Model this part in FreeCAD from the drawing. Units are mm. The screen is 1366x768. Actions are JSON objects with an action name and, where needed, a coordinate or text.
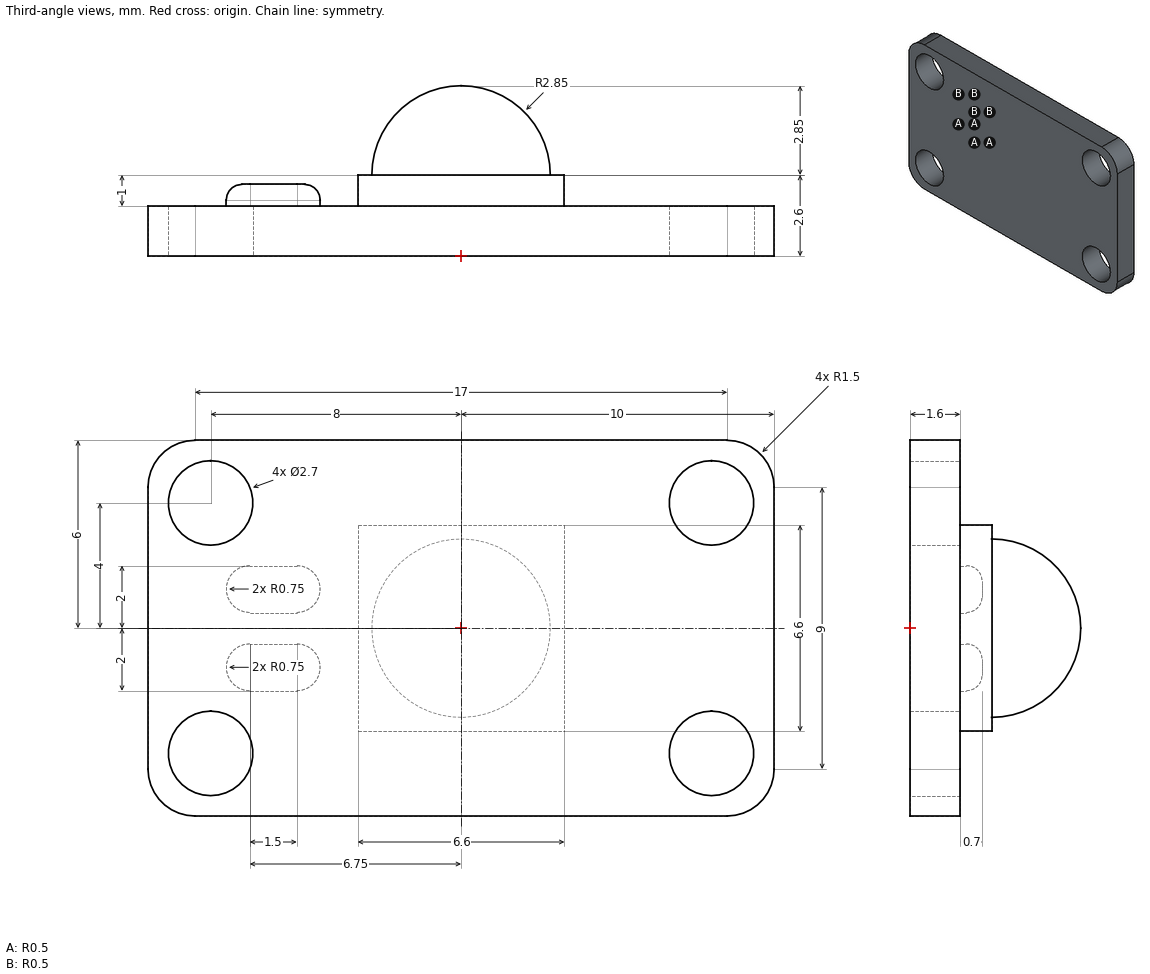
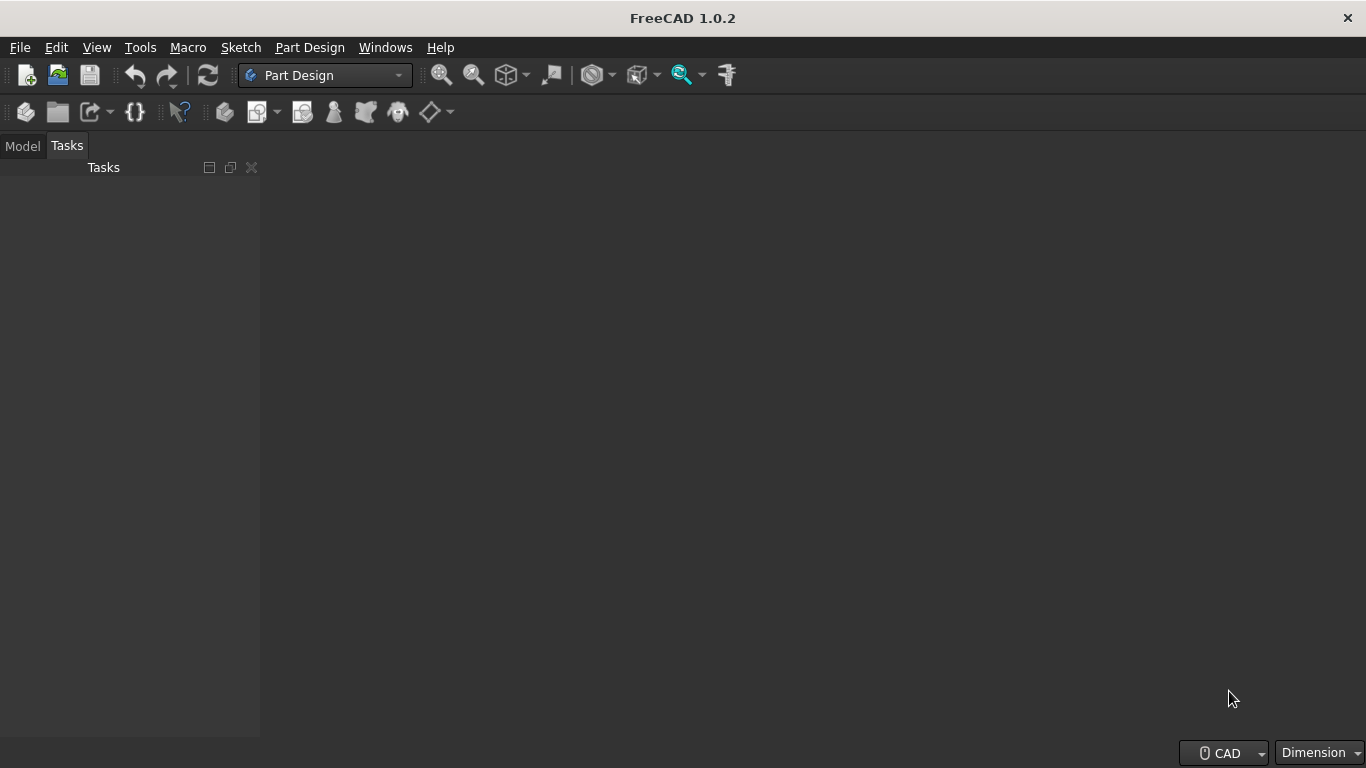
{"action": "left_click", "coordinate": [532, 112]}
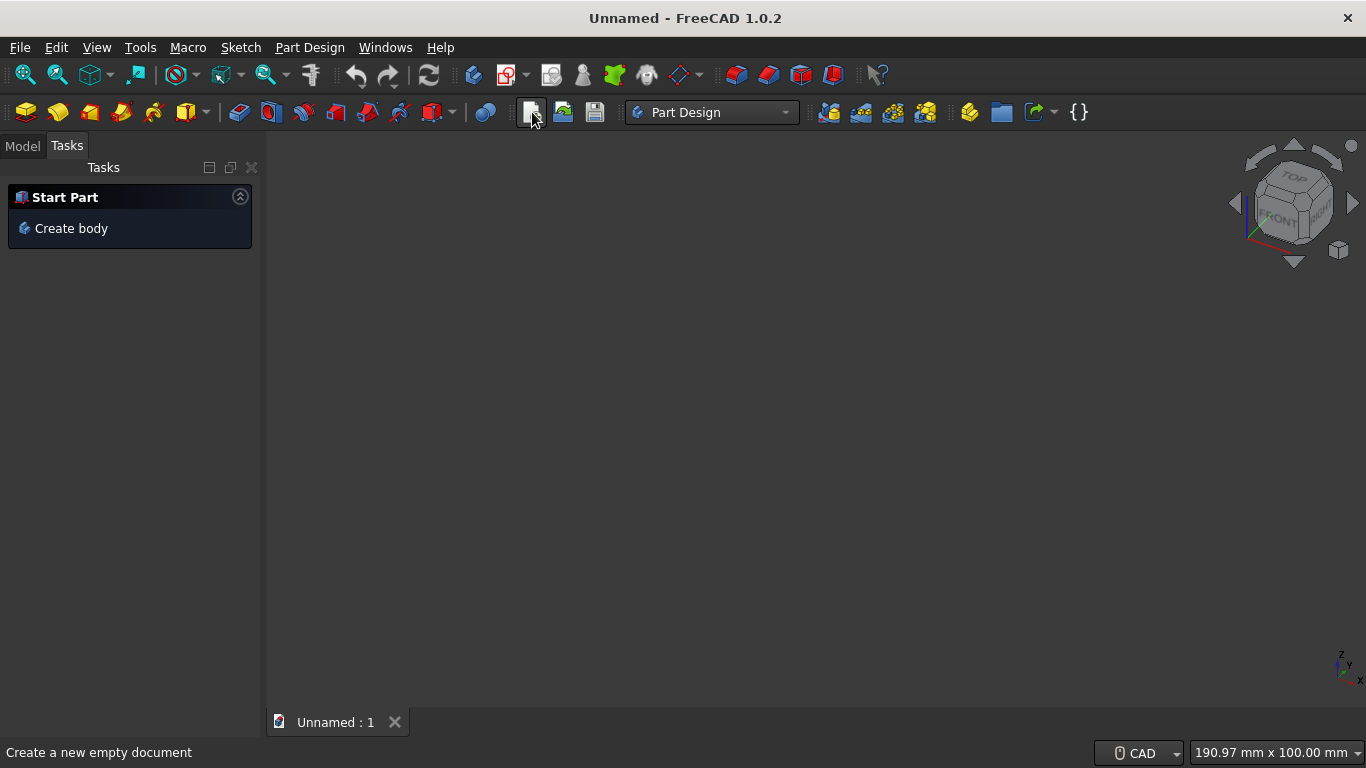
{"action": "left_click", "coordinate": [506, 76]}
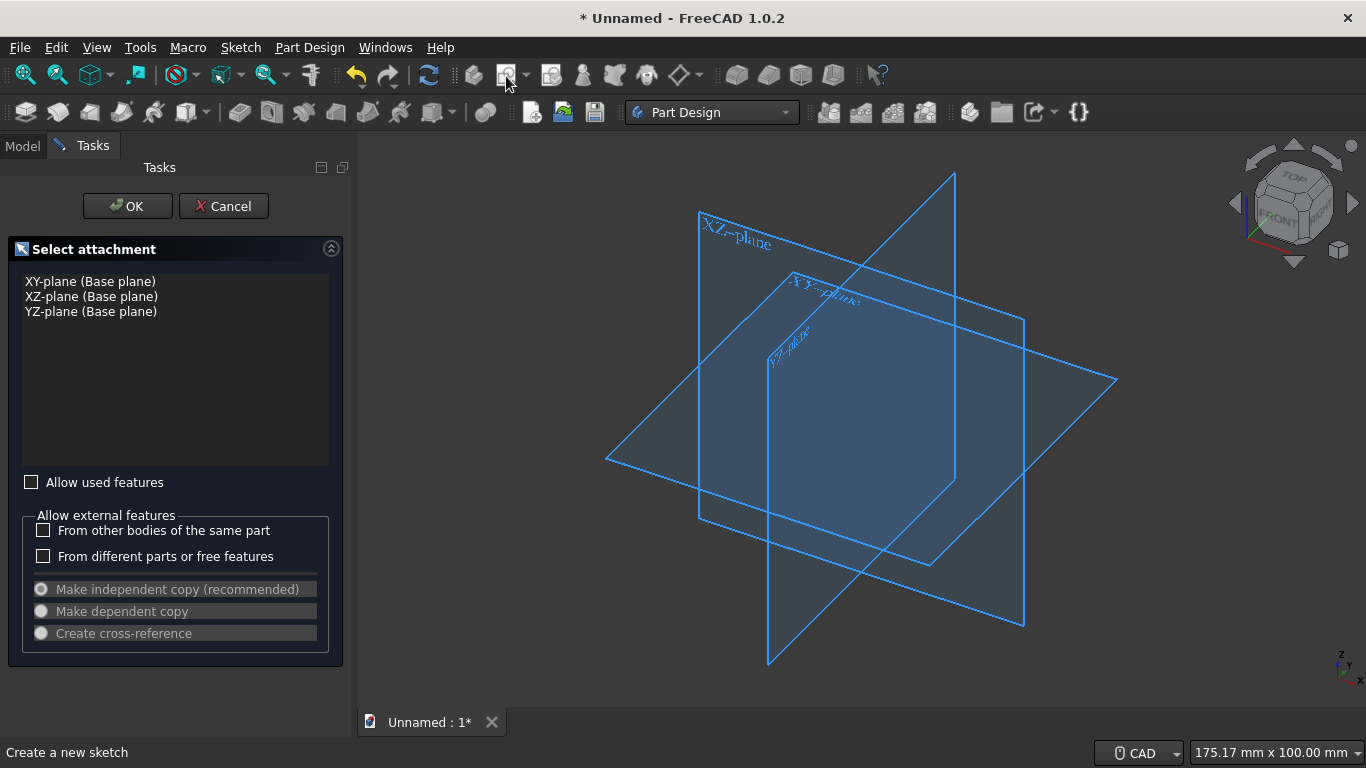
{"action": "left_click", "coordinate": [82, 296]}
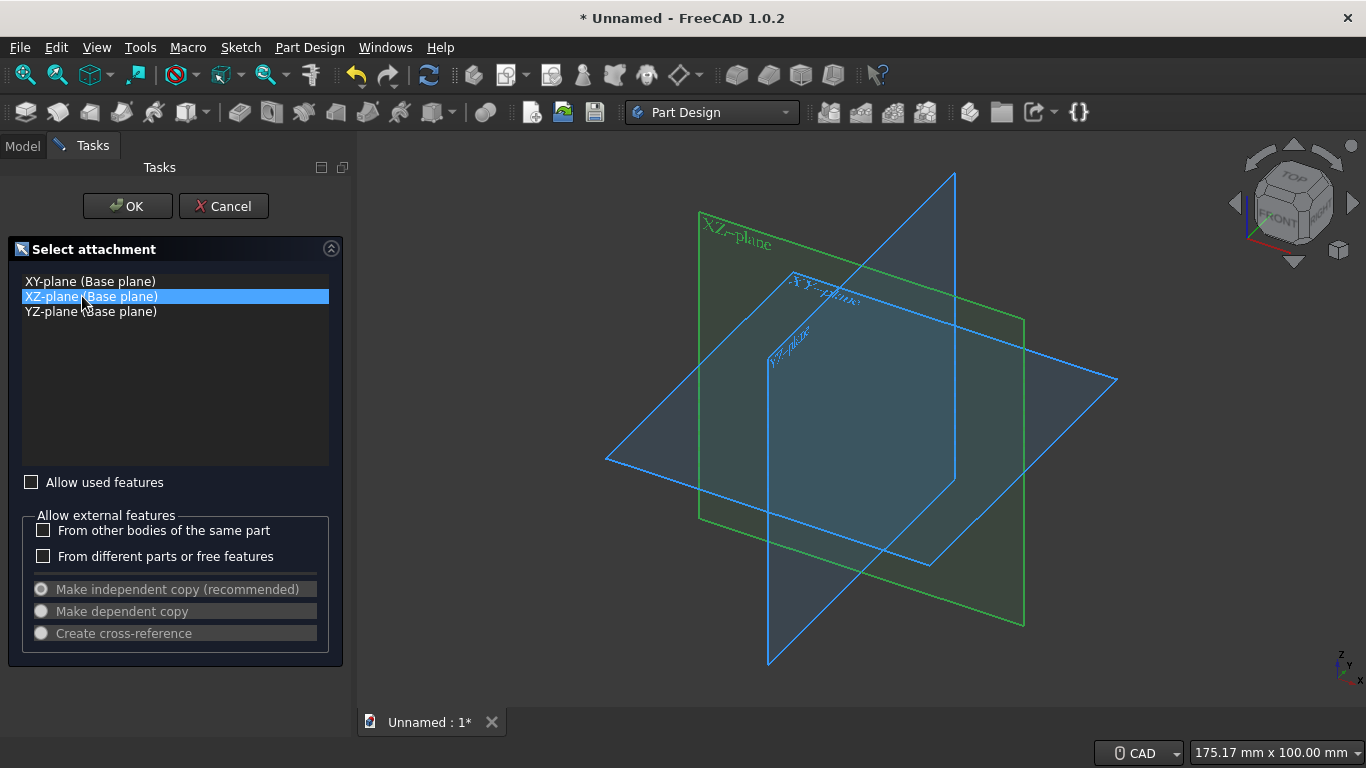
{"action": "left_click", "coordinate": [128, 206]}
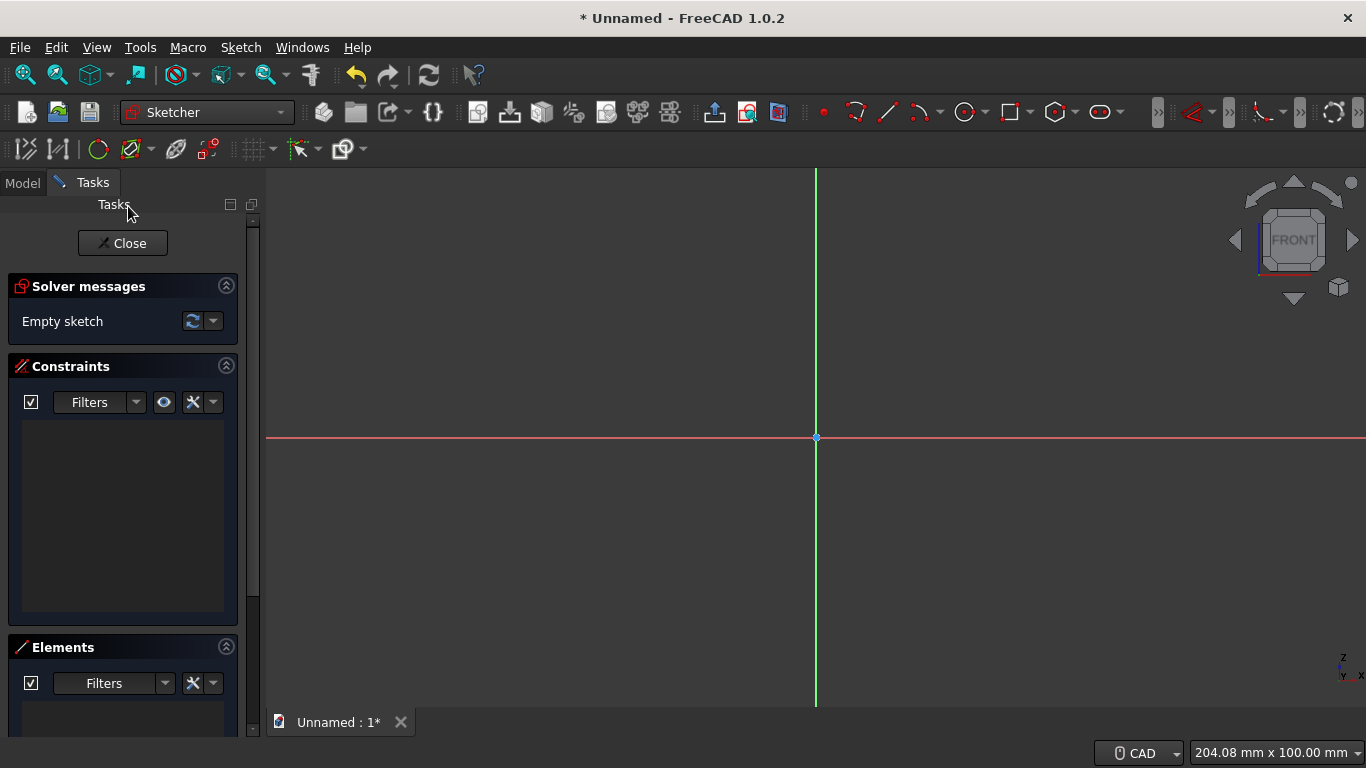
{"action": "scroll", "coordinate": [833, 438], "scroll_direction": "up", "scroll_amount": 8}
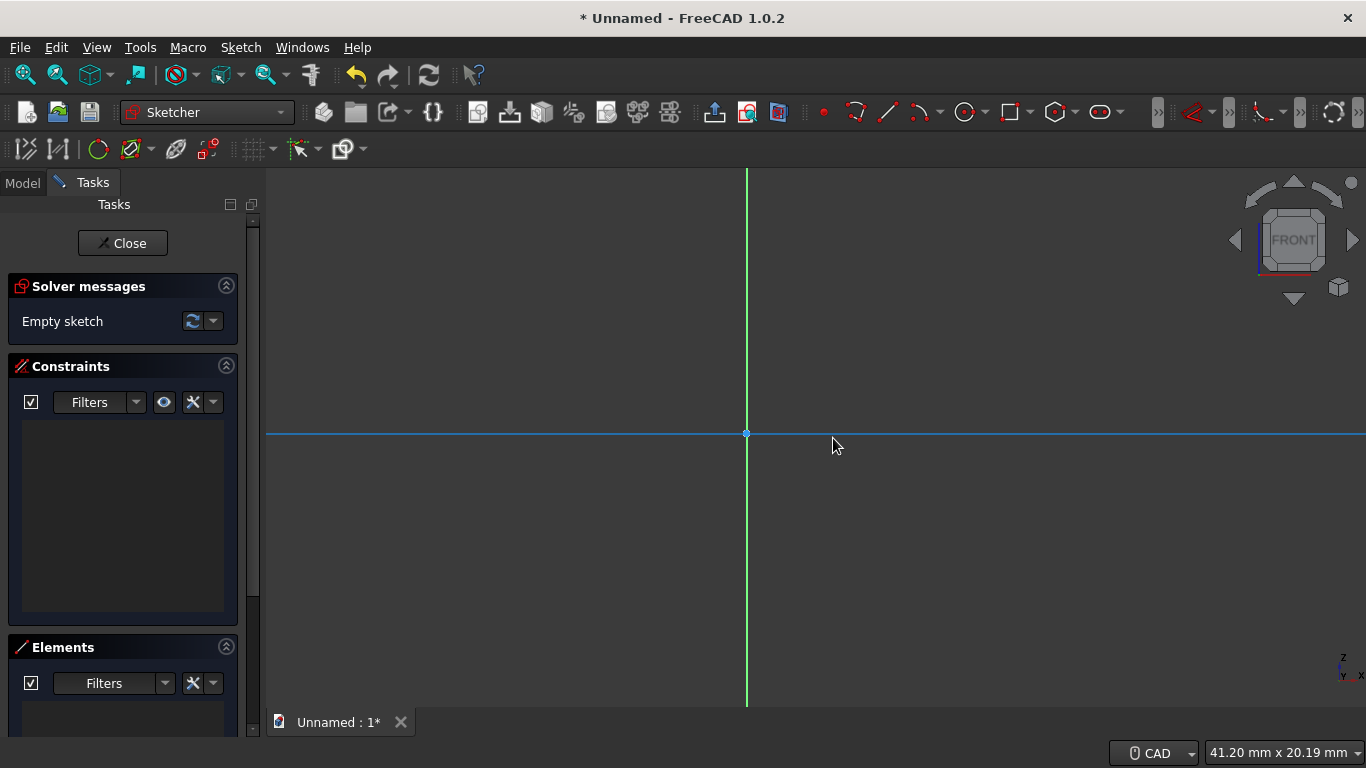
{"action": "left_click", "coordinate": [888, 112]}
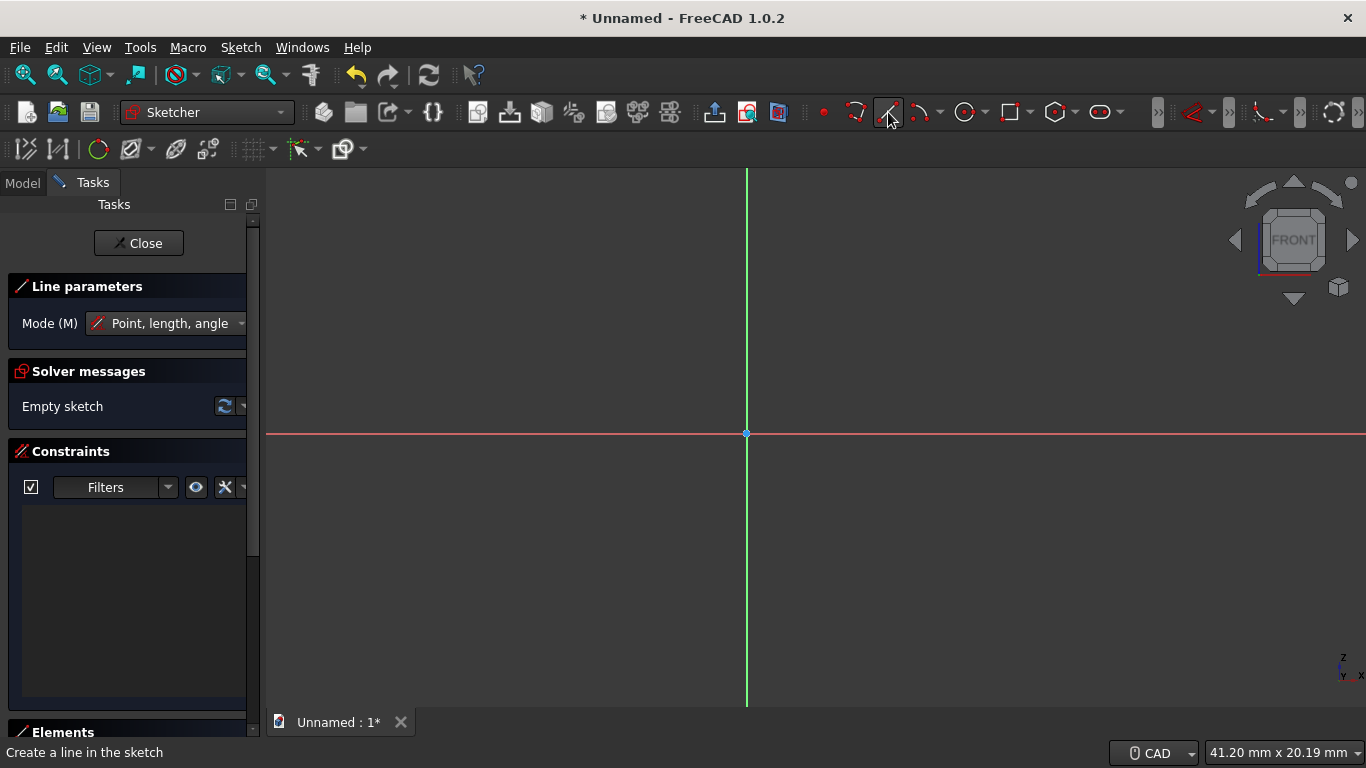
{"action": "left_click", "coordinate": [520, 273]}
{"action": "left_click", "coordinate": [974, 273]}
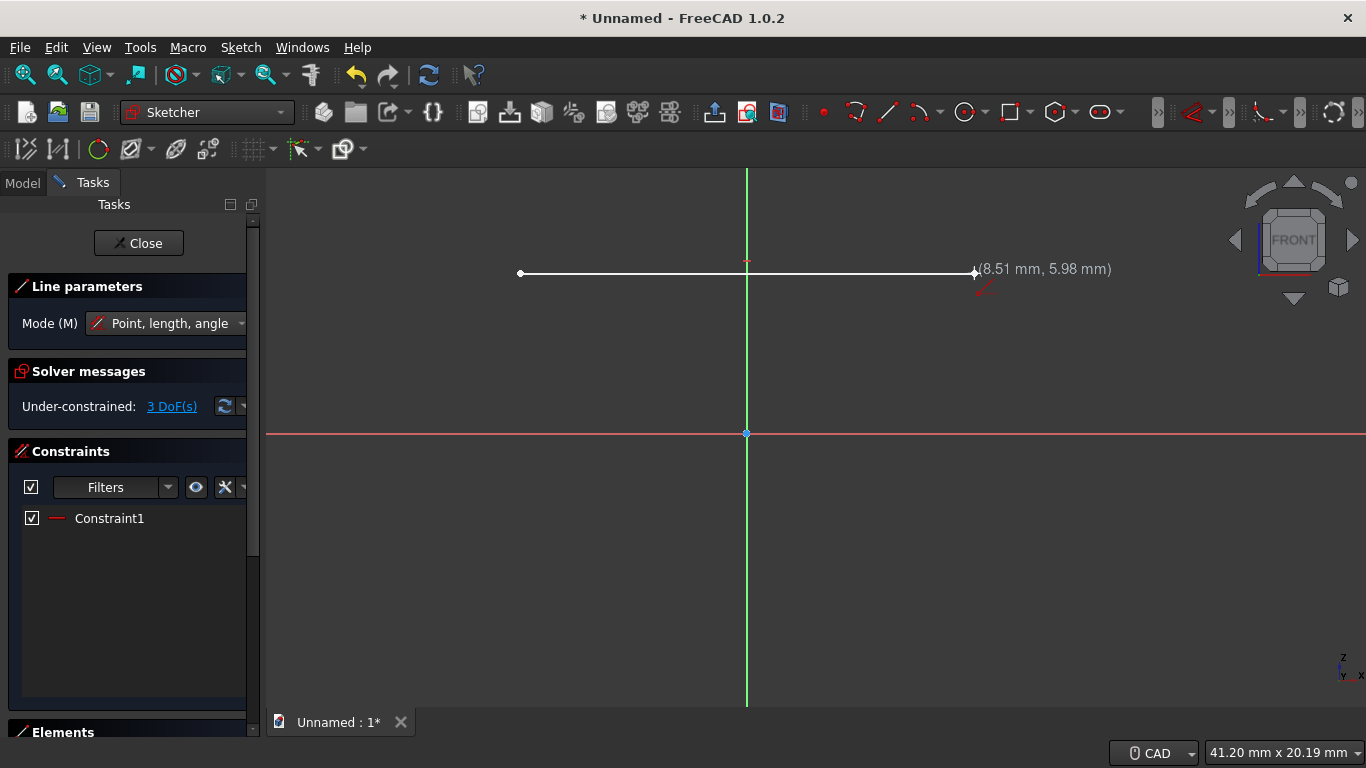
{"action": "left_click", "coordinate": [1014, 313]}
{"action": "left_click", "coordinate": [1014, 554]}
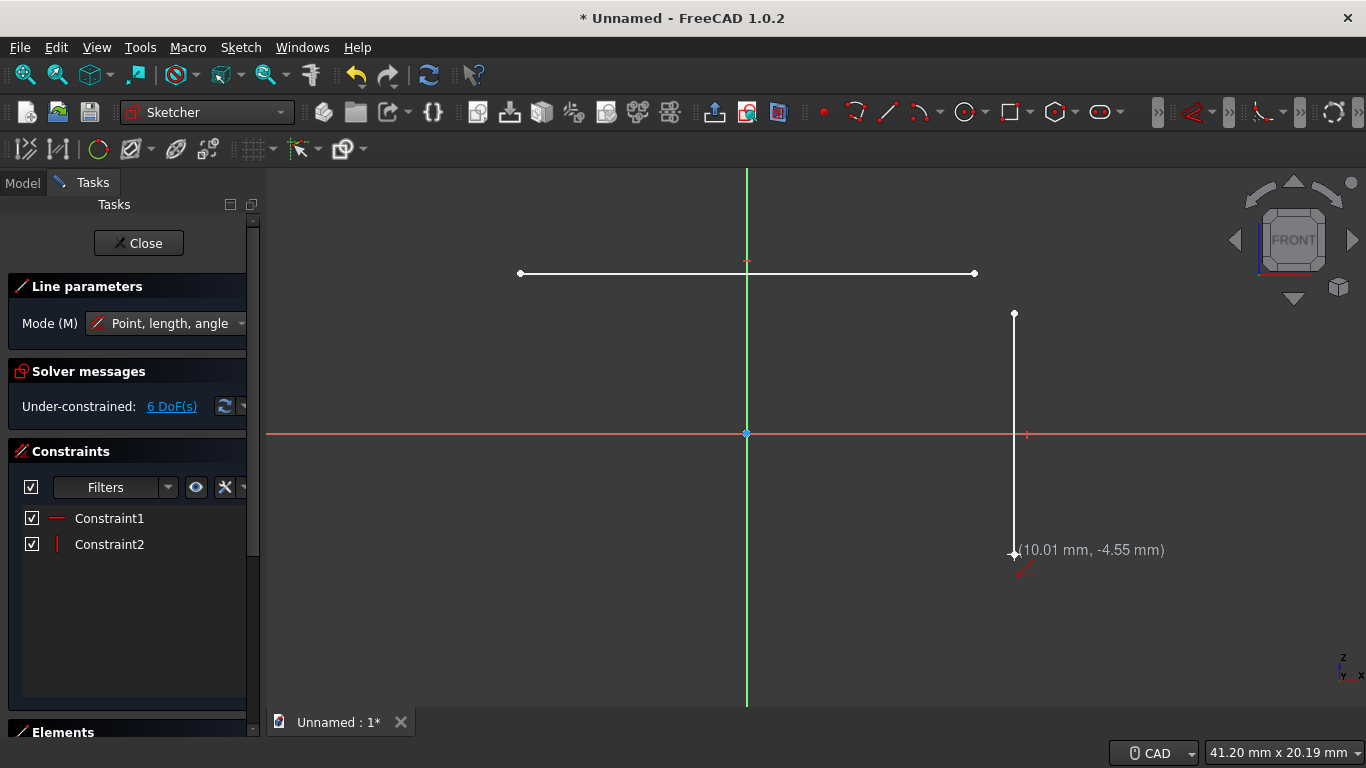
{"action": "left_click", "coordinate": [974, 594]}
{"action": "left_click", "coordinate": [520, 594]}